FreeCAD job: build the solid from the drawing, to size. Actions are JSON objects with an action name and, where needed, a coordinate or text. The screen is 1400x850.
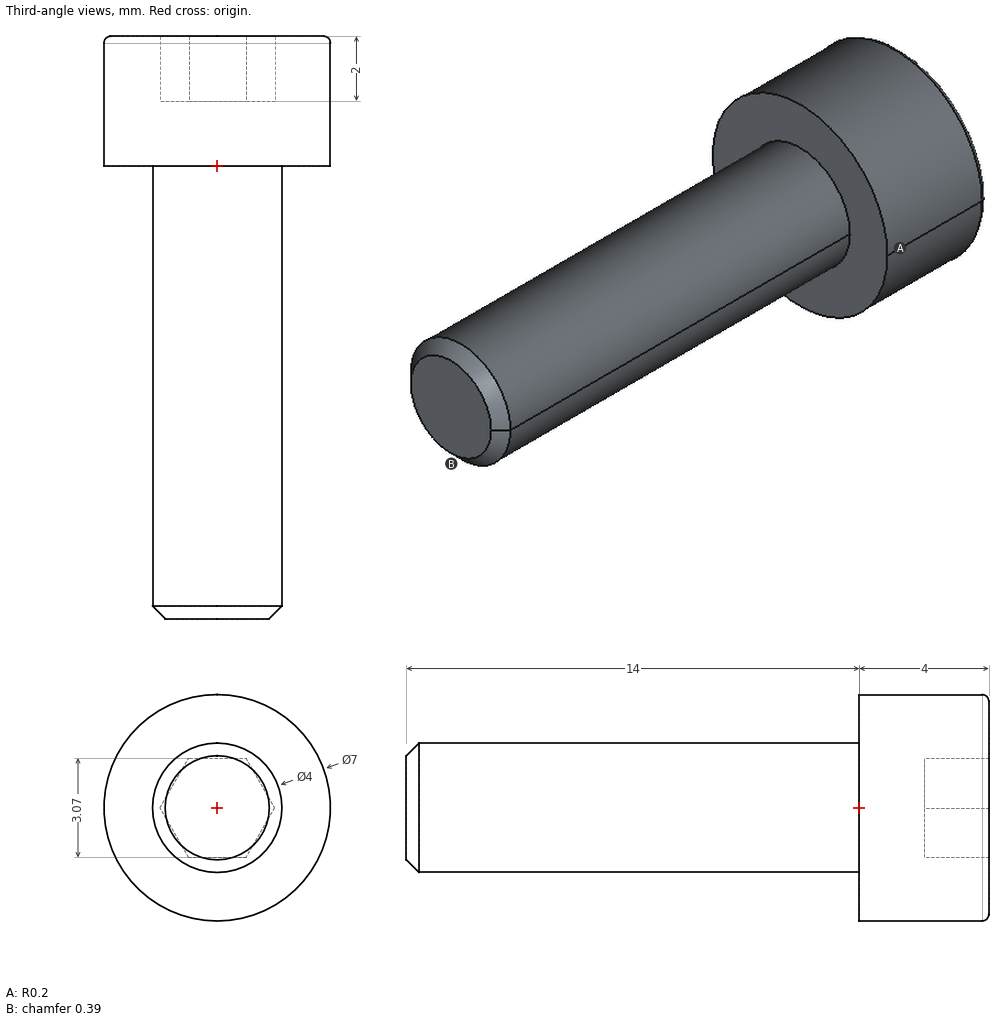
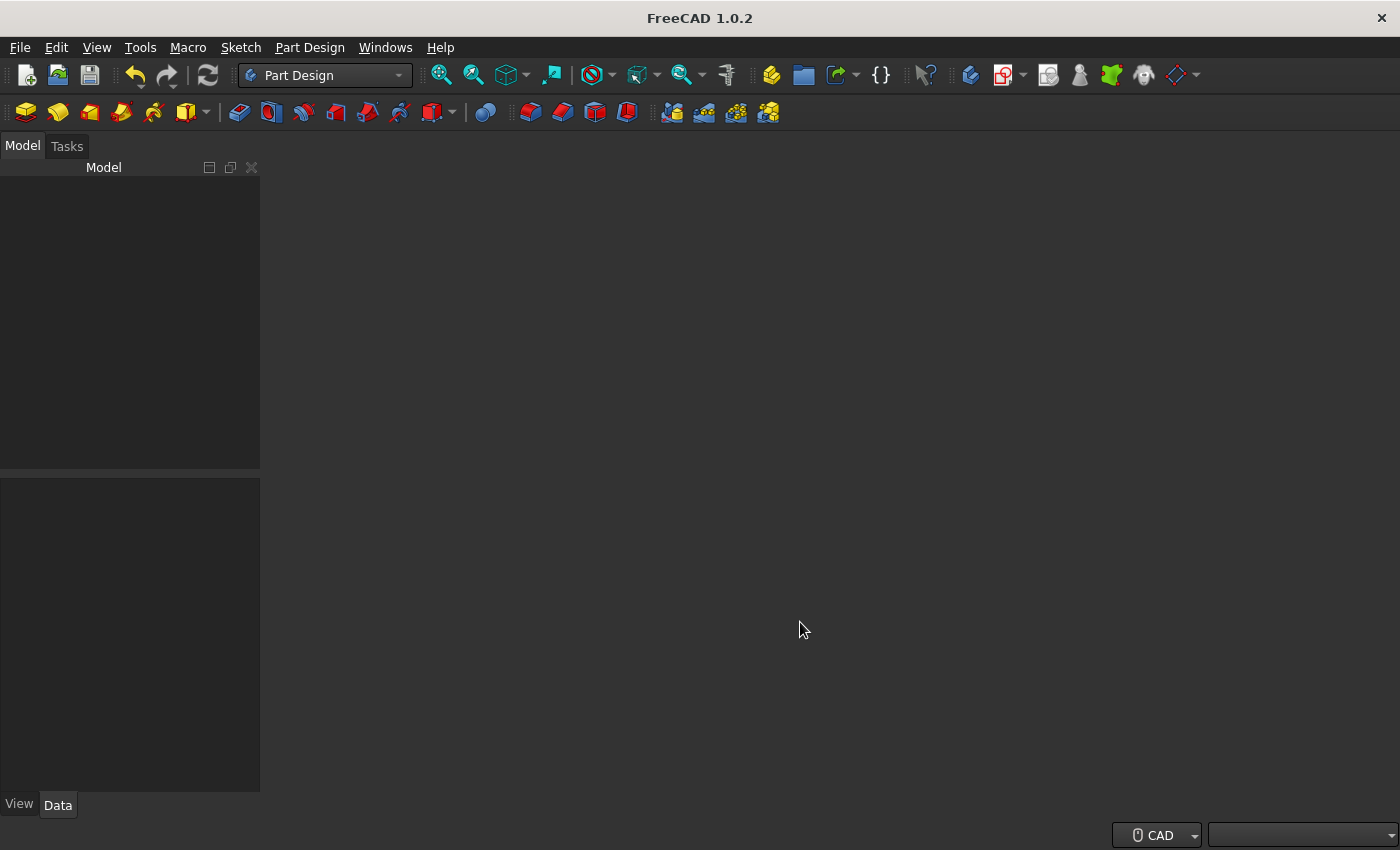
{"action": "left_click", "coordinate": [26, 76]}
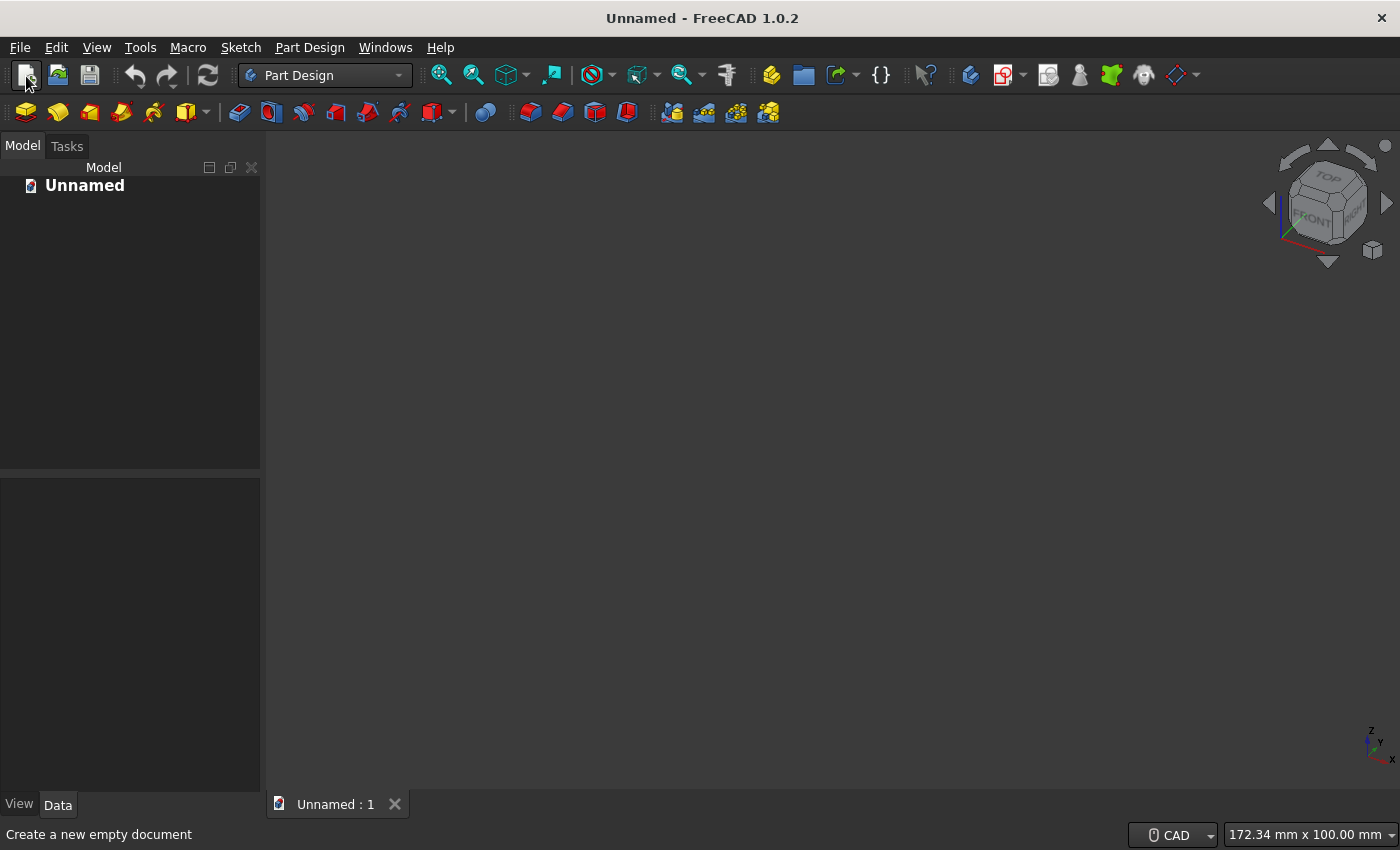
{"action": "left_click", "coordinate": [1004, 76]}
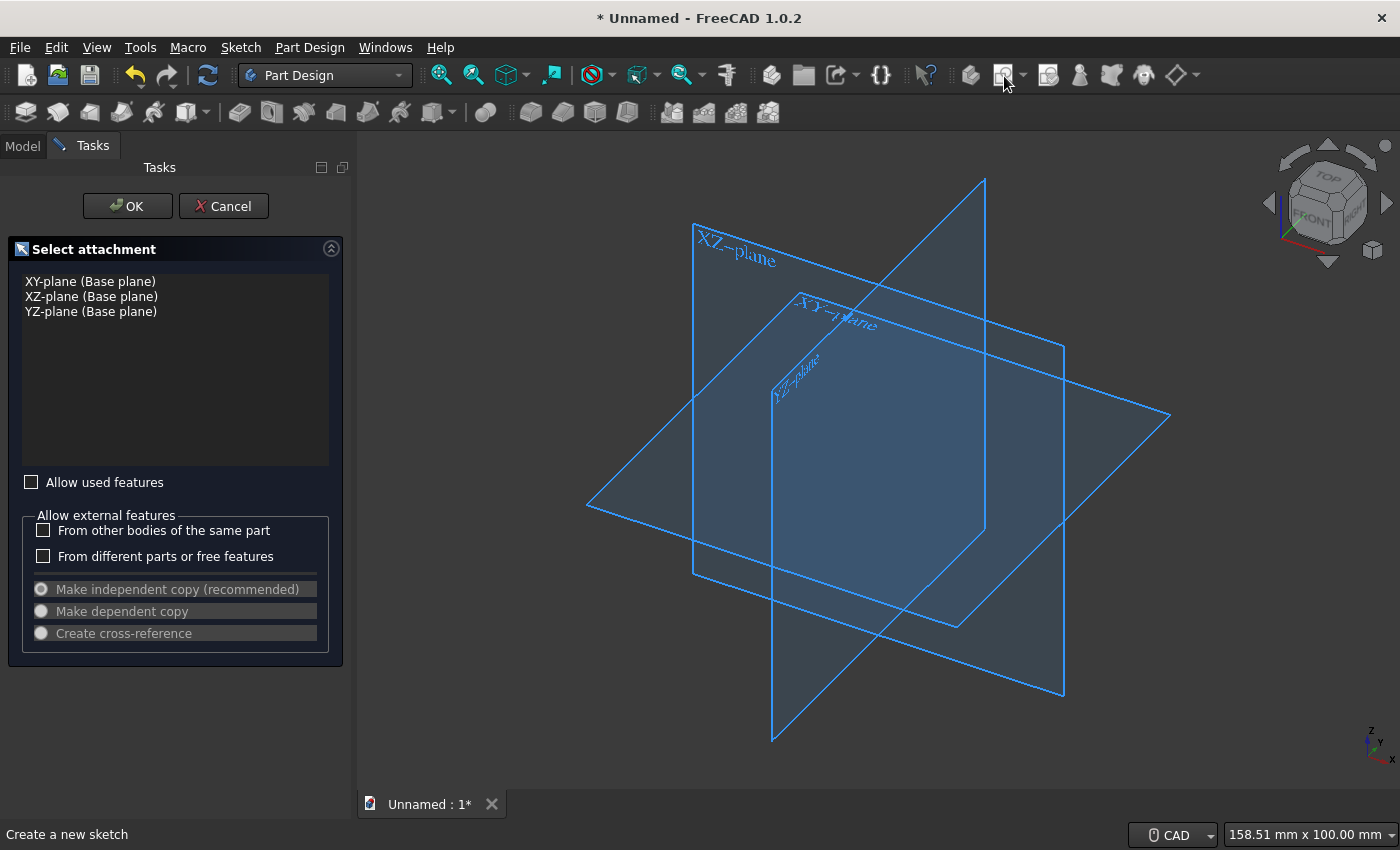
{"action": "left_click", "coordinate": [82, 296]}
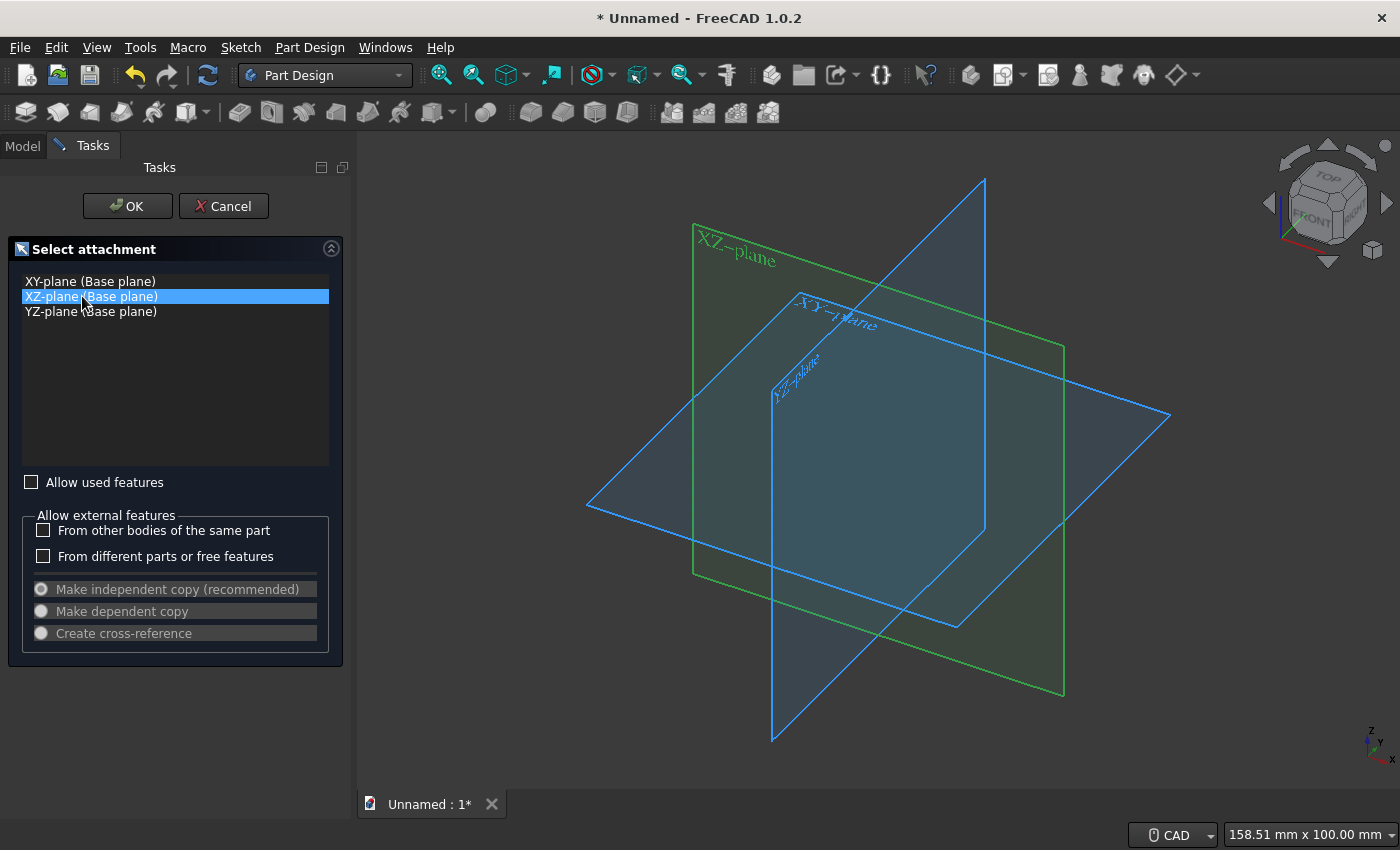
{"action": "left_click", "coordinate": [128, 206]}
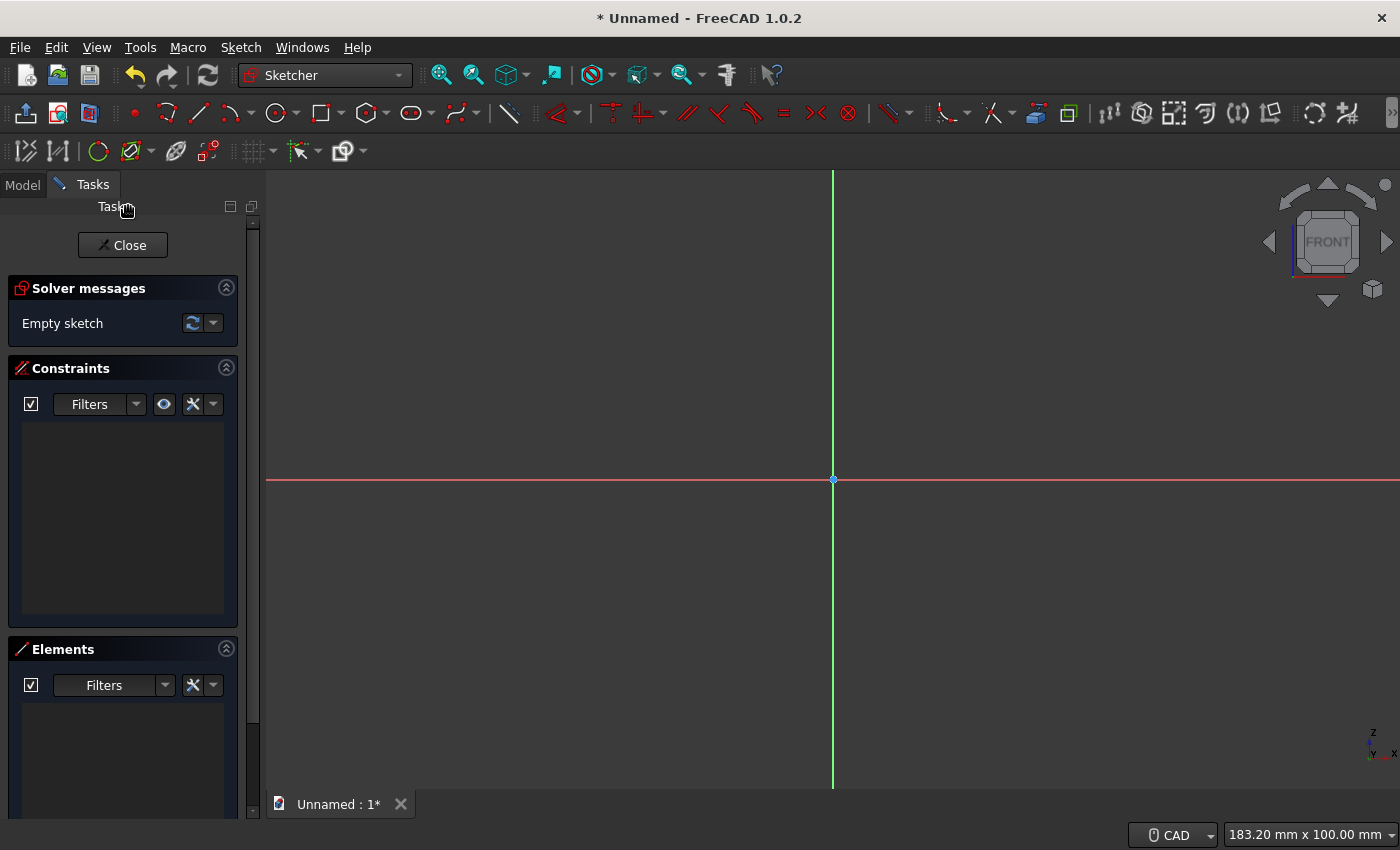
{"action": "scroll", "coordinate": [842, 479], "scroll_direction": "up", "scroll_amount": 11}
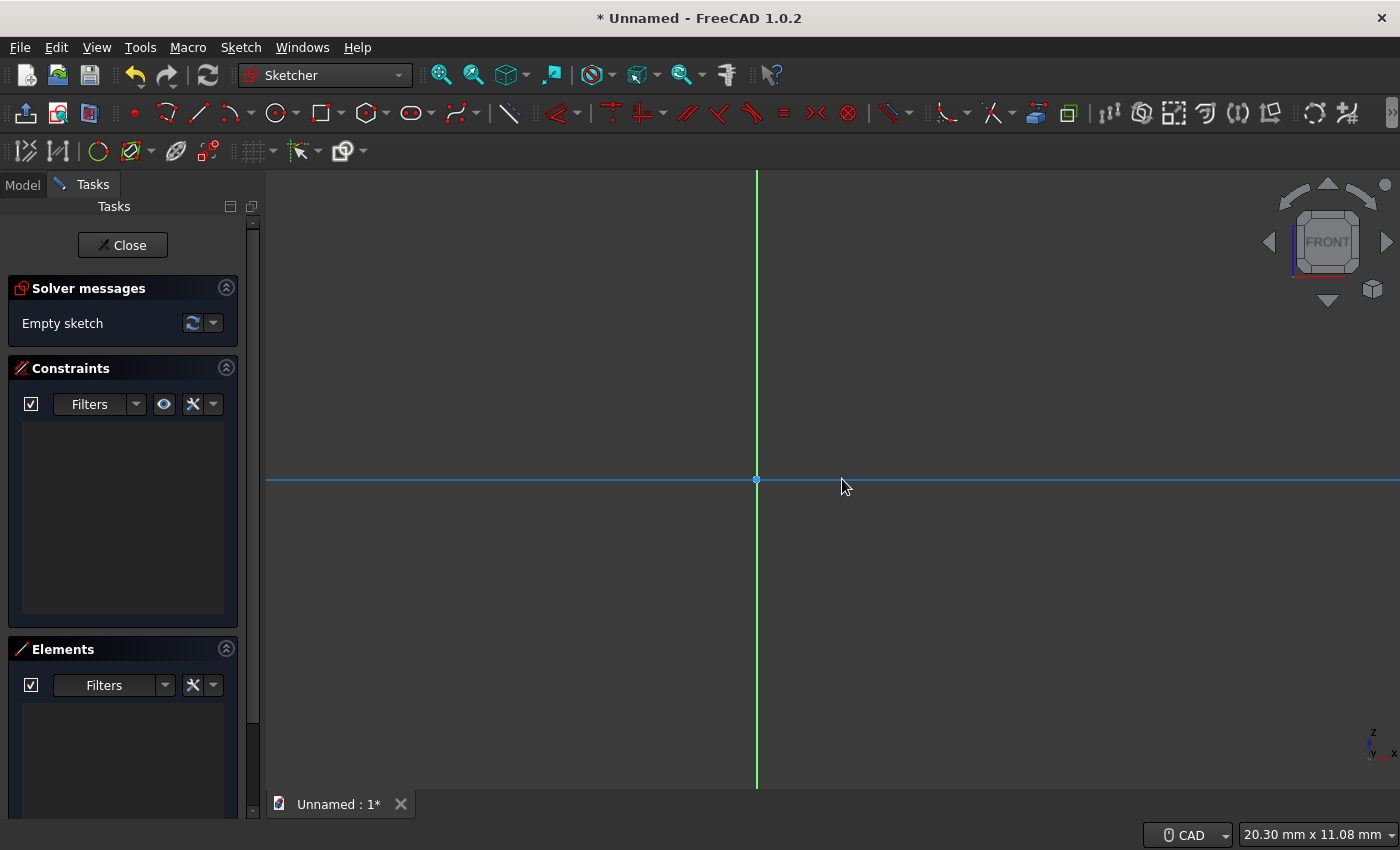
{"action": "left_click", "coordinate": [276, 114]}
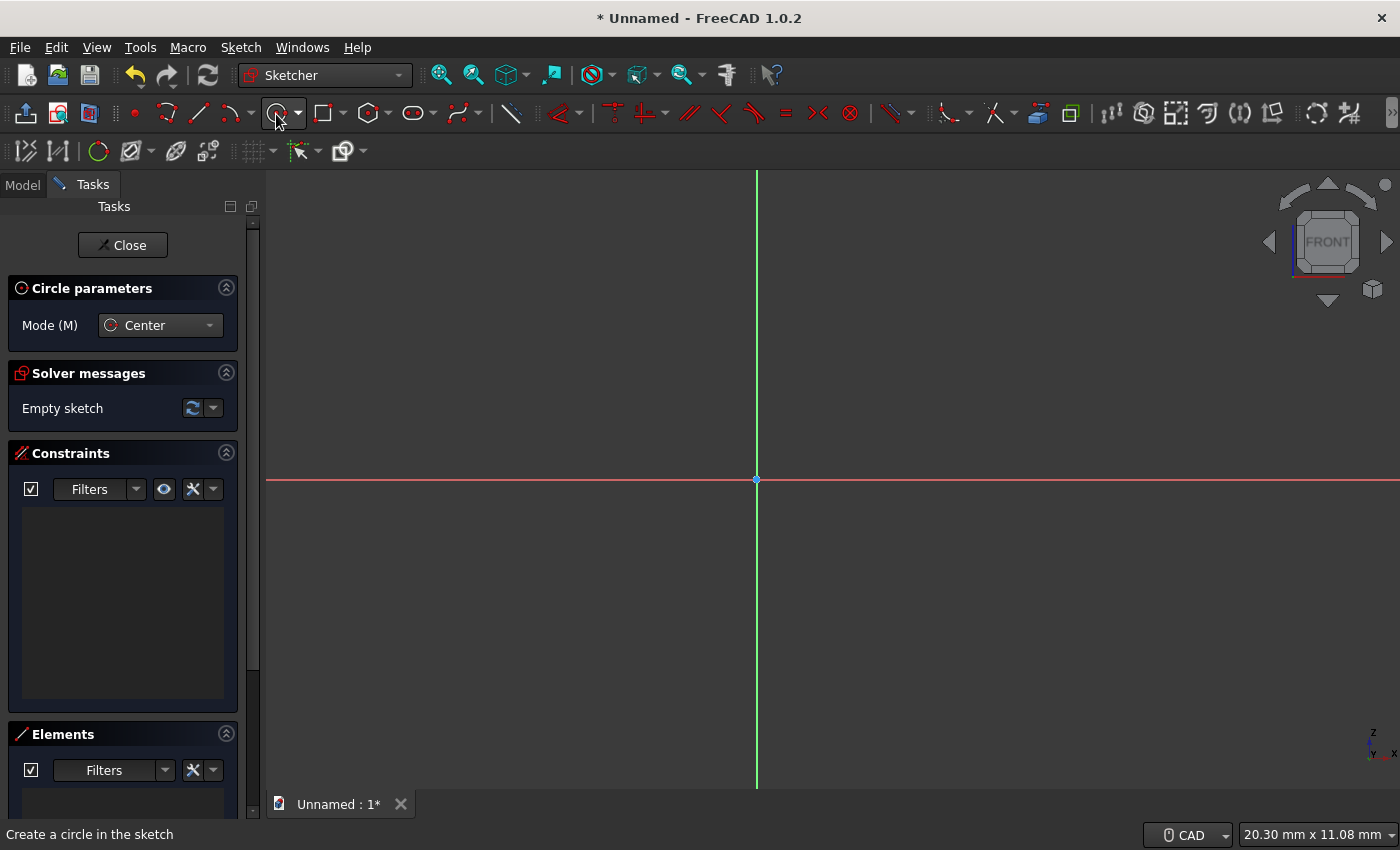
{"action": "left_click", "coordinate": [757, 480]}
{"action": "mouse_move", "coordinate": [895, 341]}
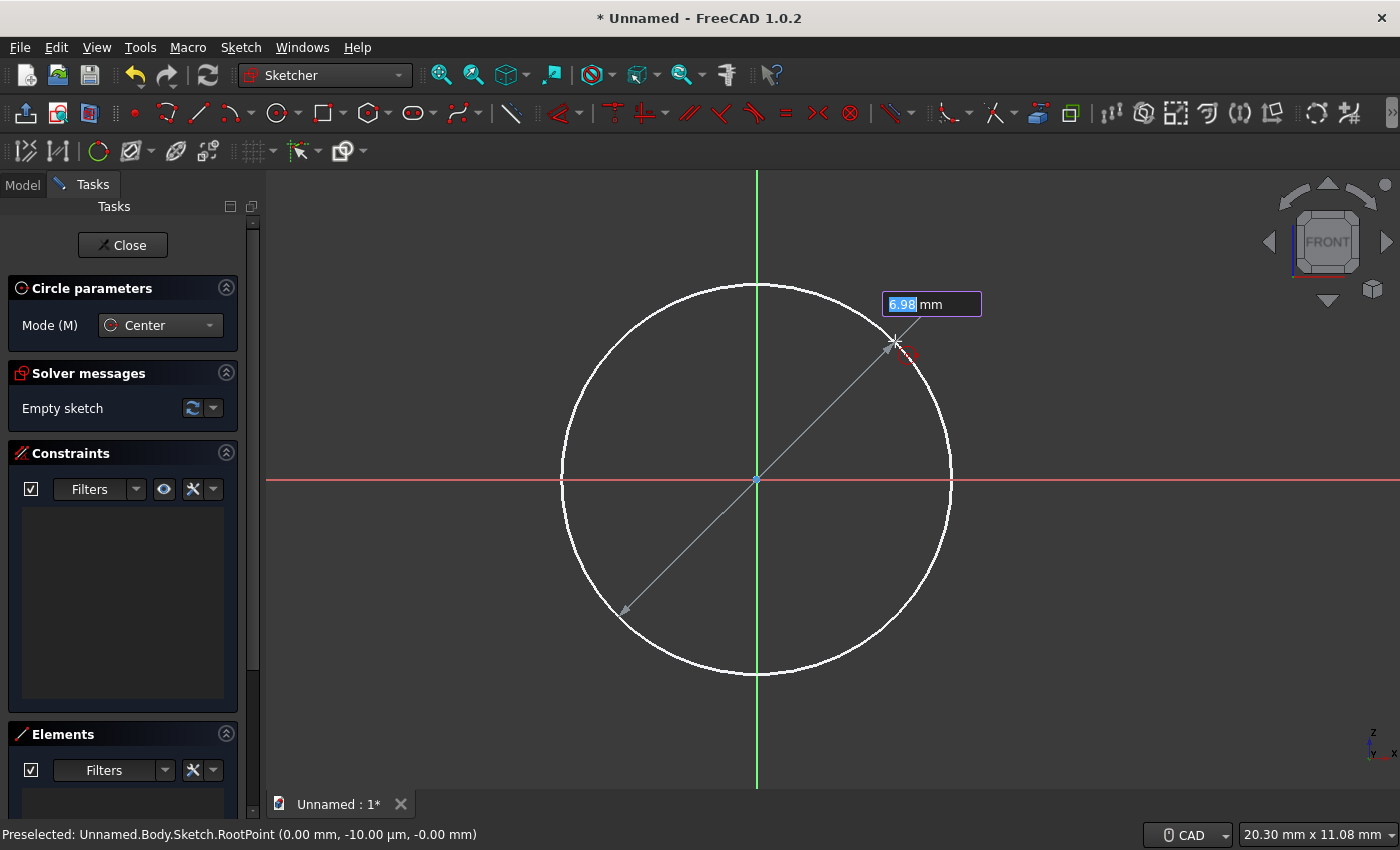
{"action": "type", "text": "7"}
{"action": "key", "text": "Return"}
{"action": "key", "text": "Escape"}